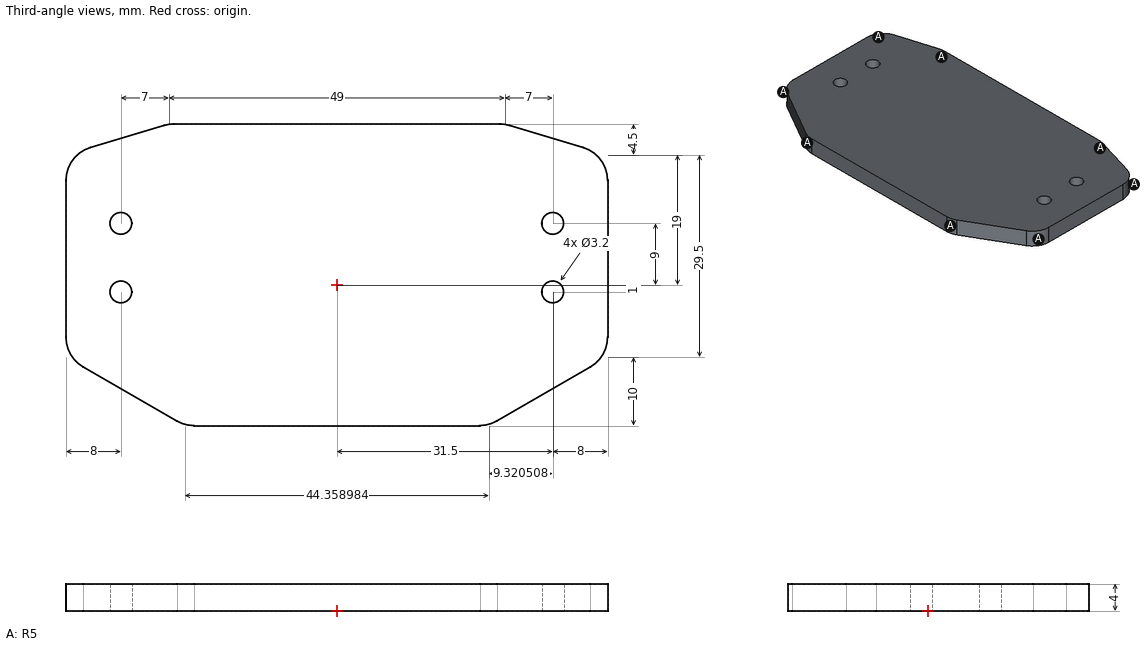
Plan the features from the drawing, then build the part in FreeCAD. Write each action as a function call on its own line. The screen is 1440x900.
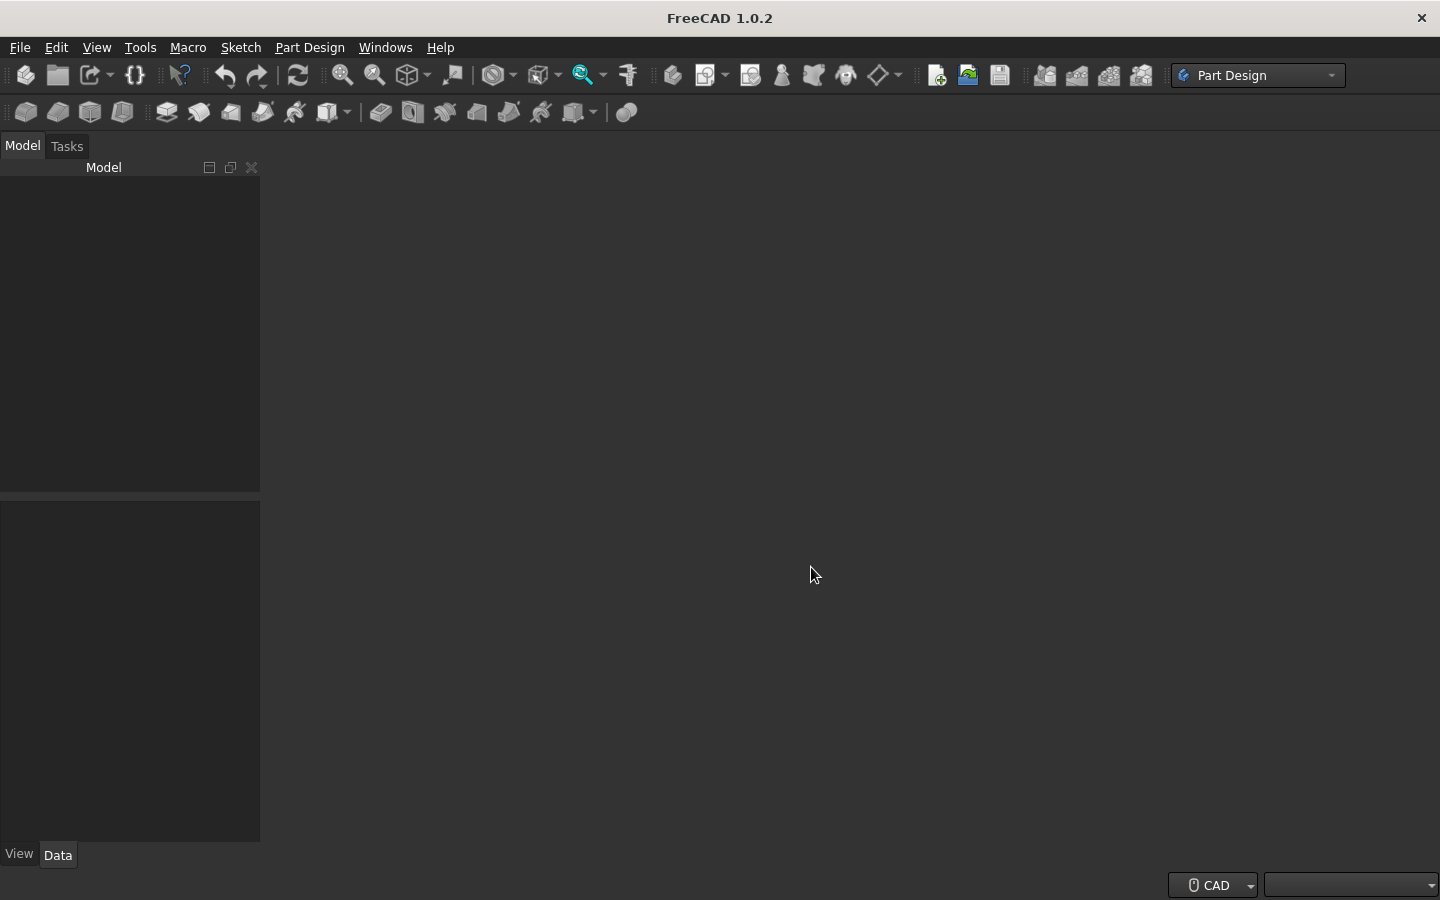
click(936, 76)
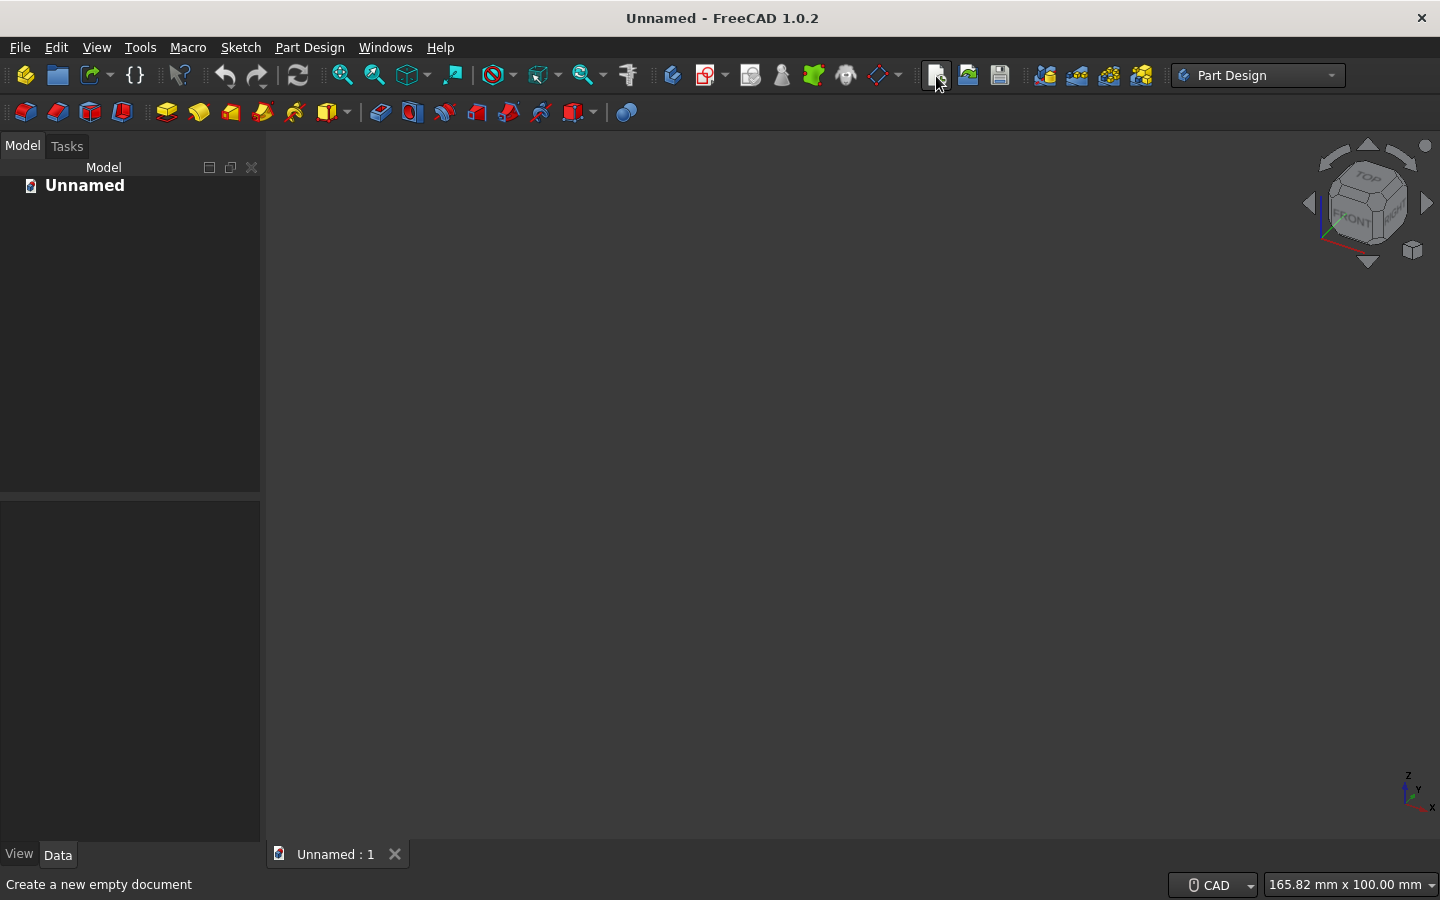
click(706, 76)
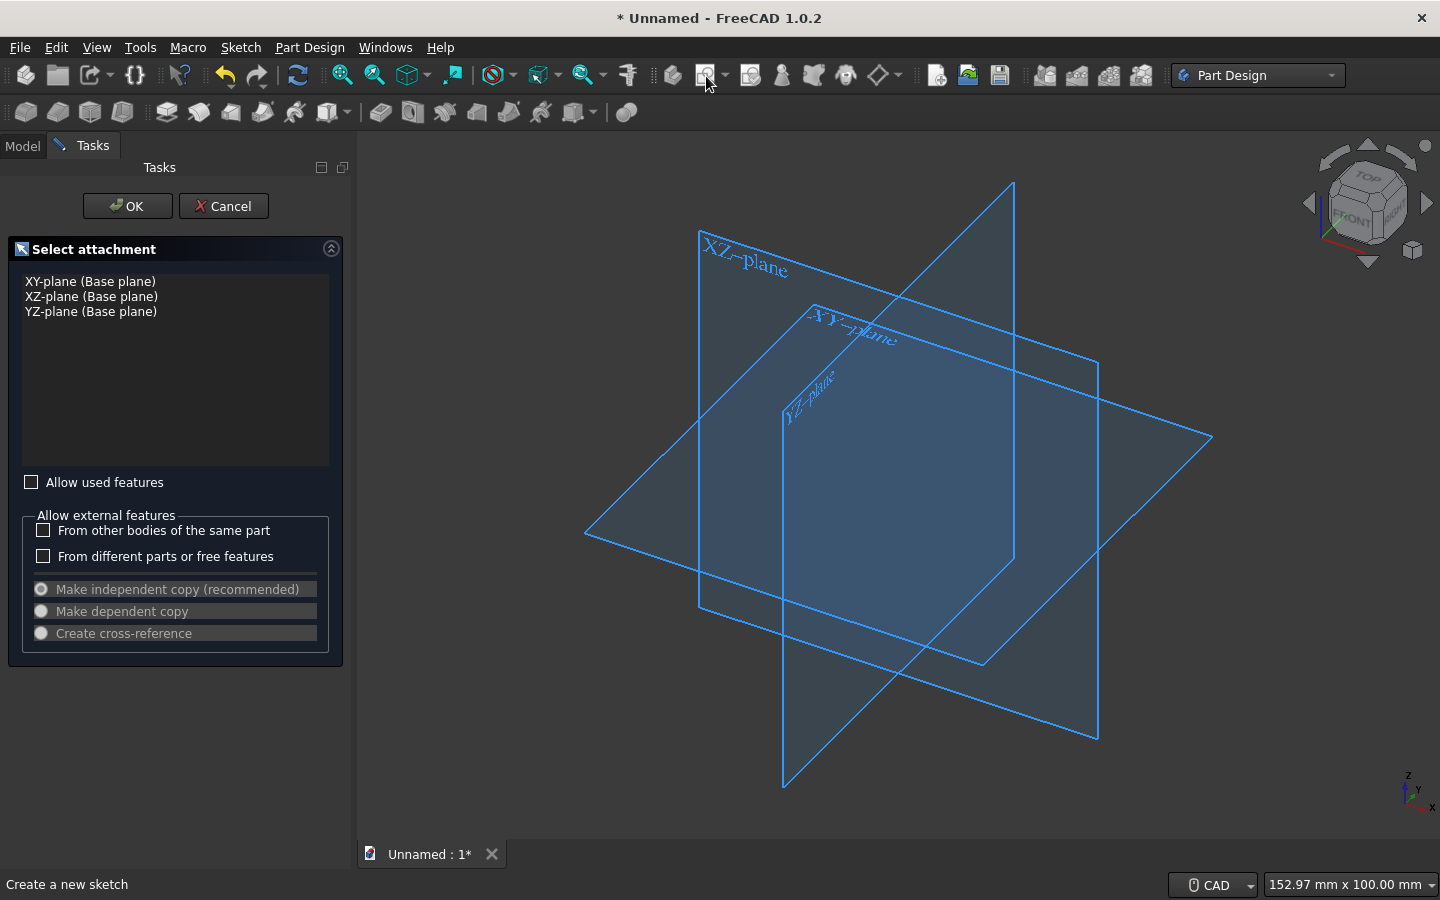
click(82, 282)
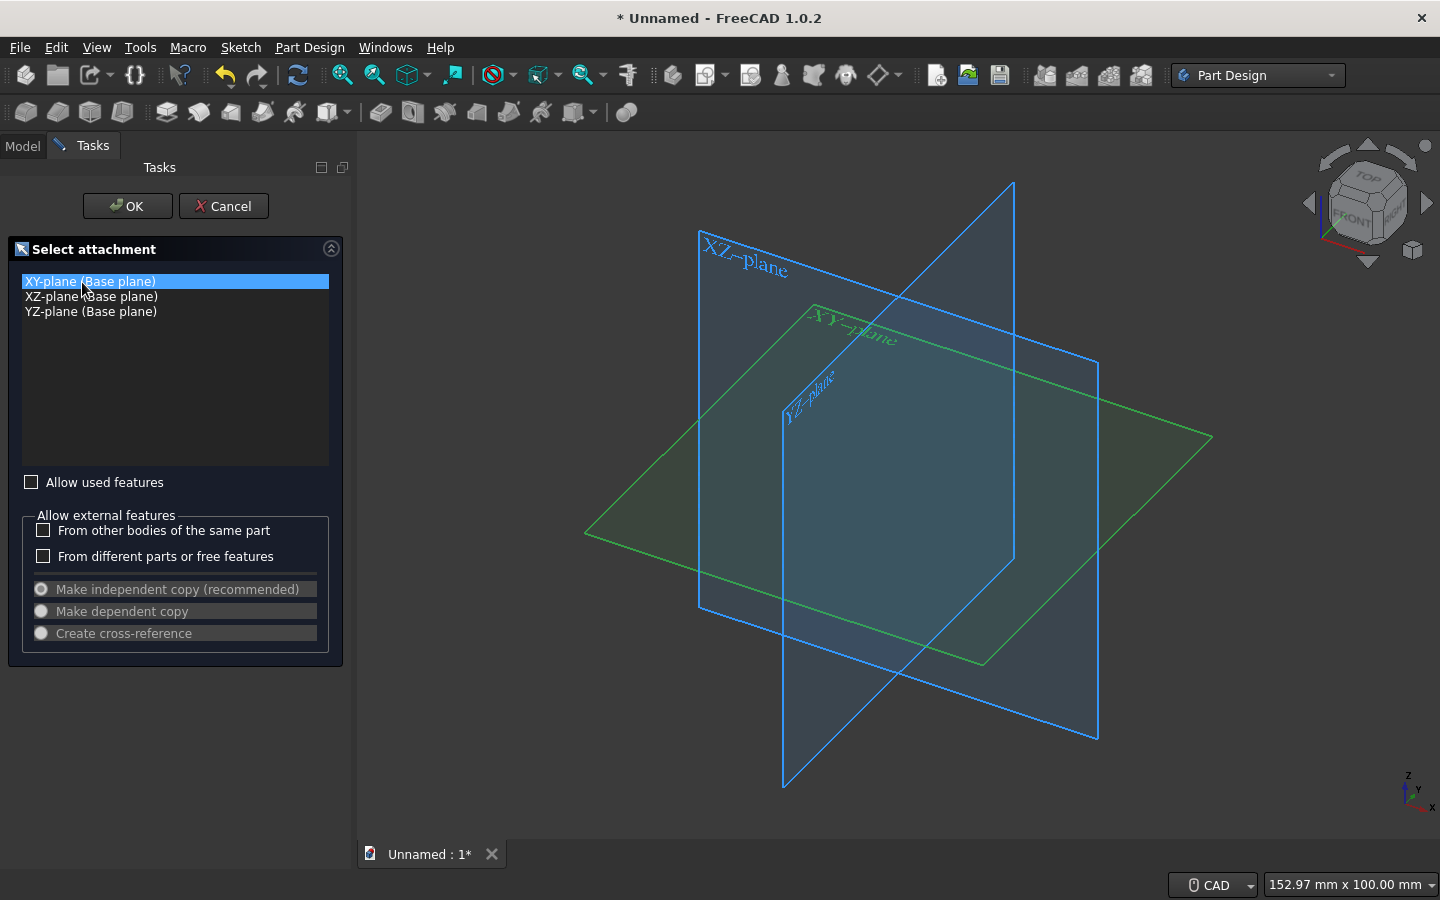
click(128, 206)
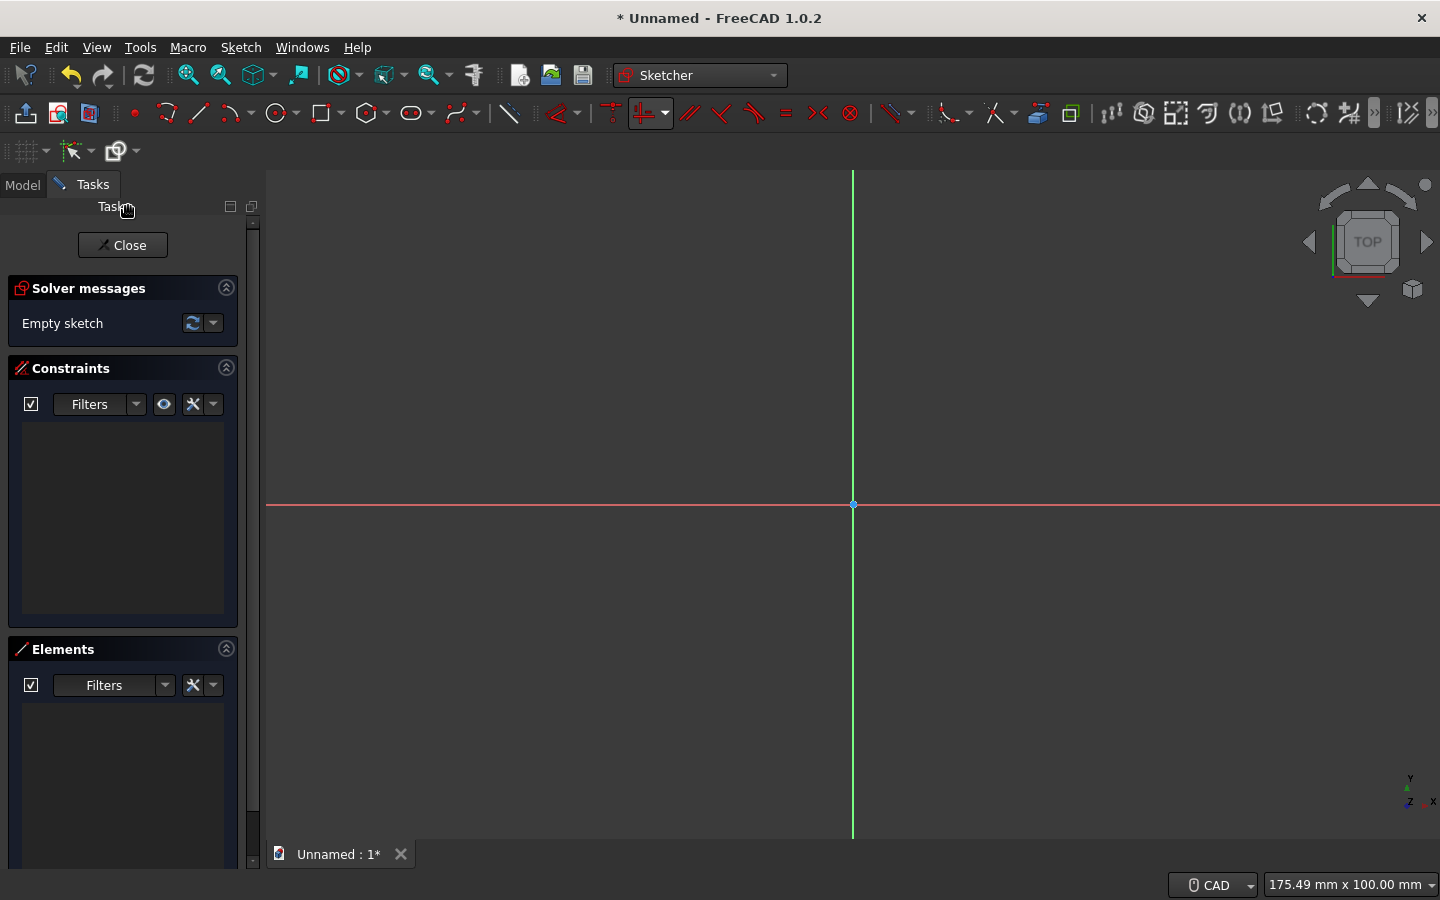
click(168, 114)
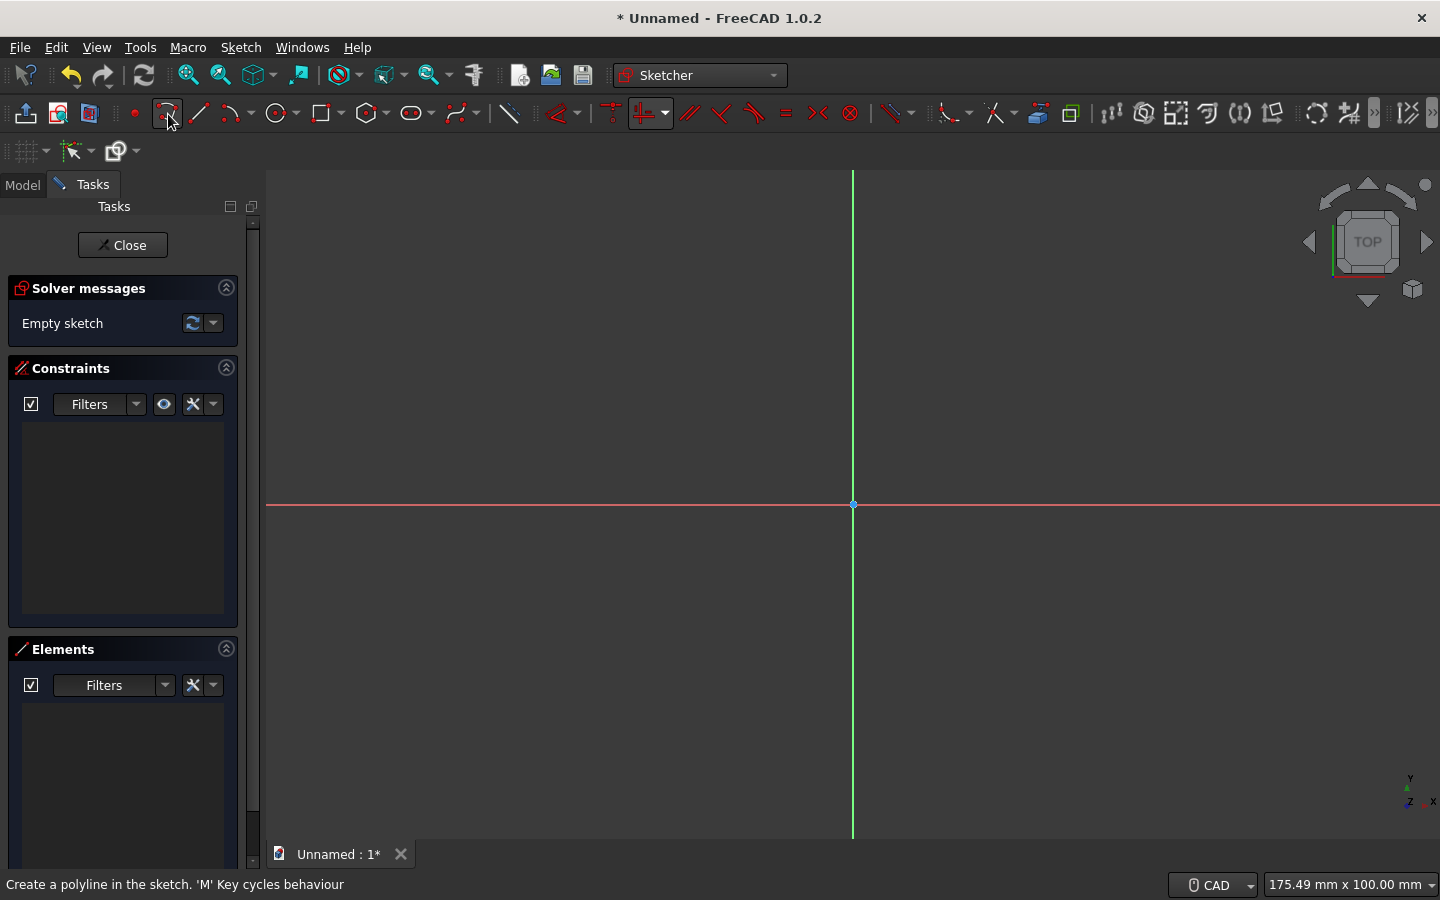
click(705, 642)
click(1001, 642)
click(1117, 575)
click(1117, 377)
click(1017, 347)
click(689, 347)
click(589, 377)
click(589, 575)
click(705, 643)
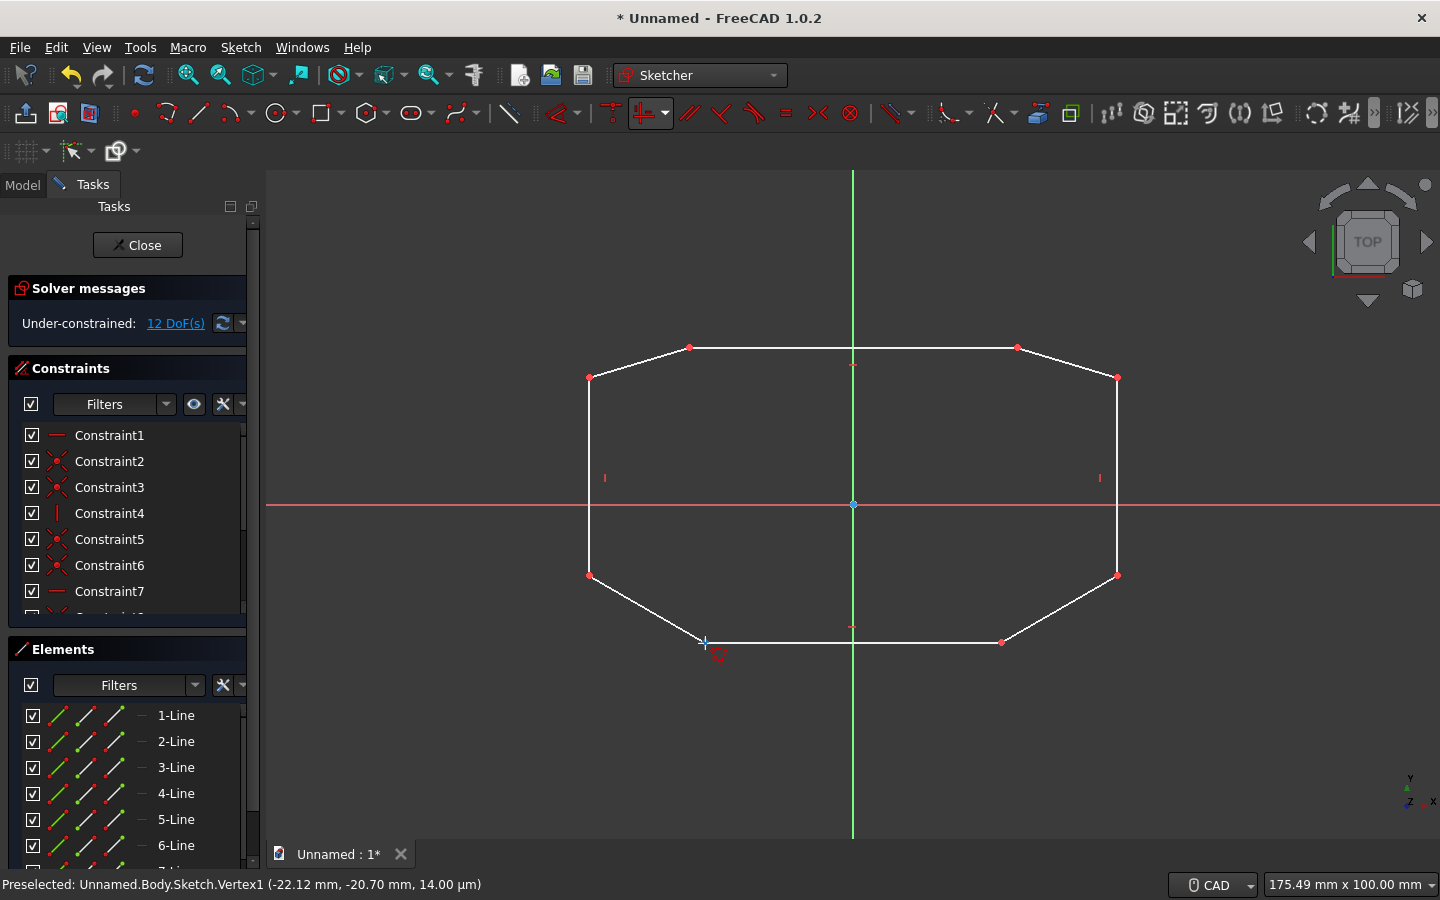
key(g)
key(c)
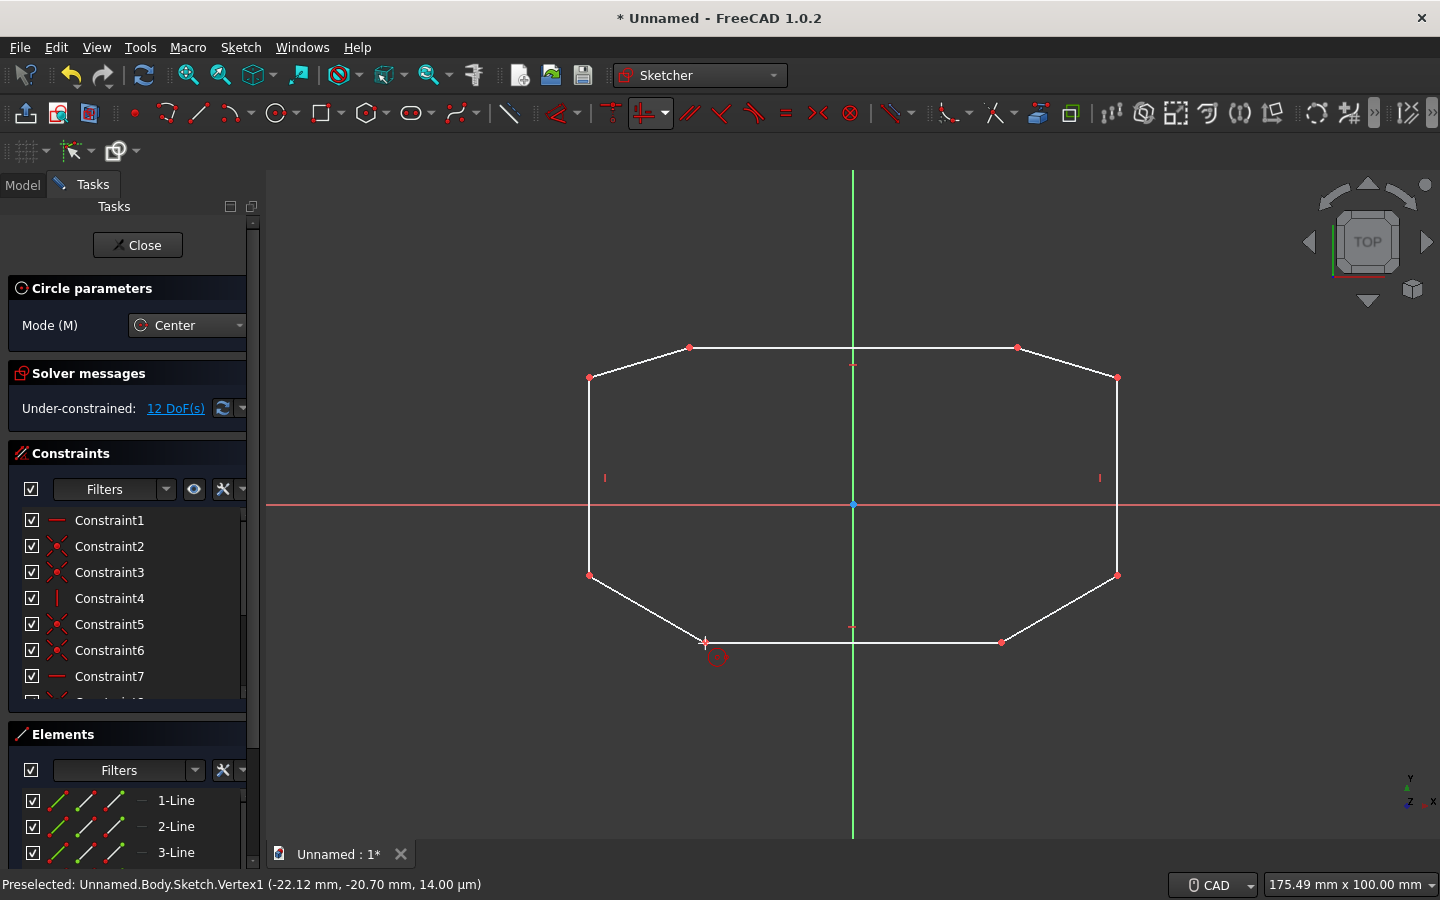
scroll(1064, 511, up, 5)